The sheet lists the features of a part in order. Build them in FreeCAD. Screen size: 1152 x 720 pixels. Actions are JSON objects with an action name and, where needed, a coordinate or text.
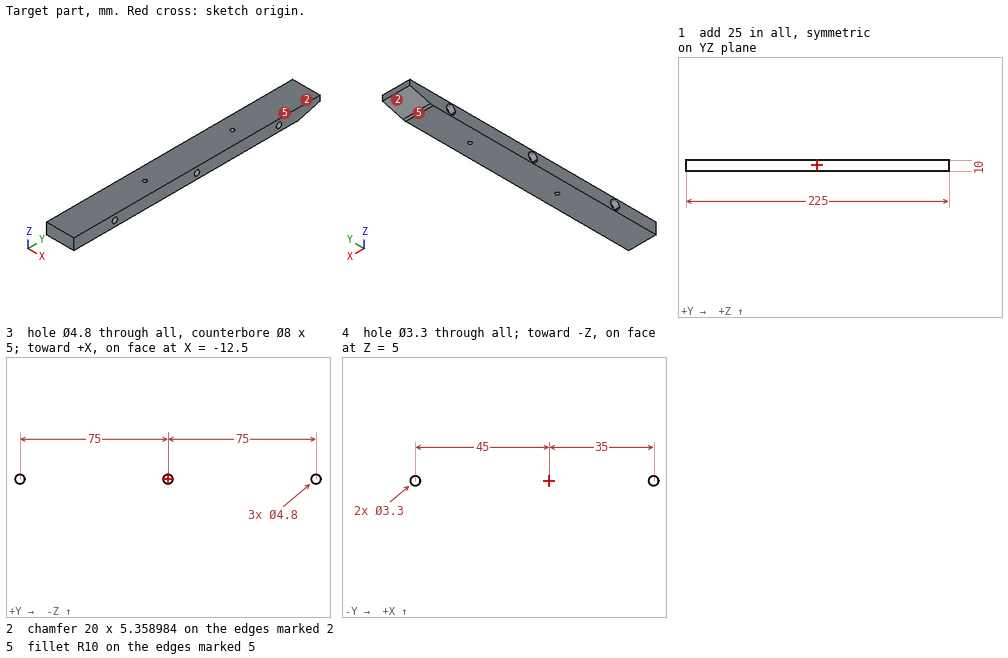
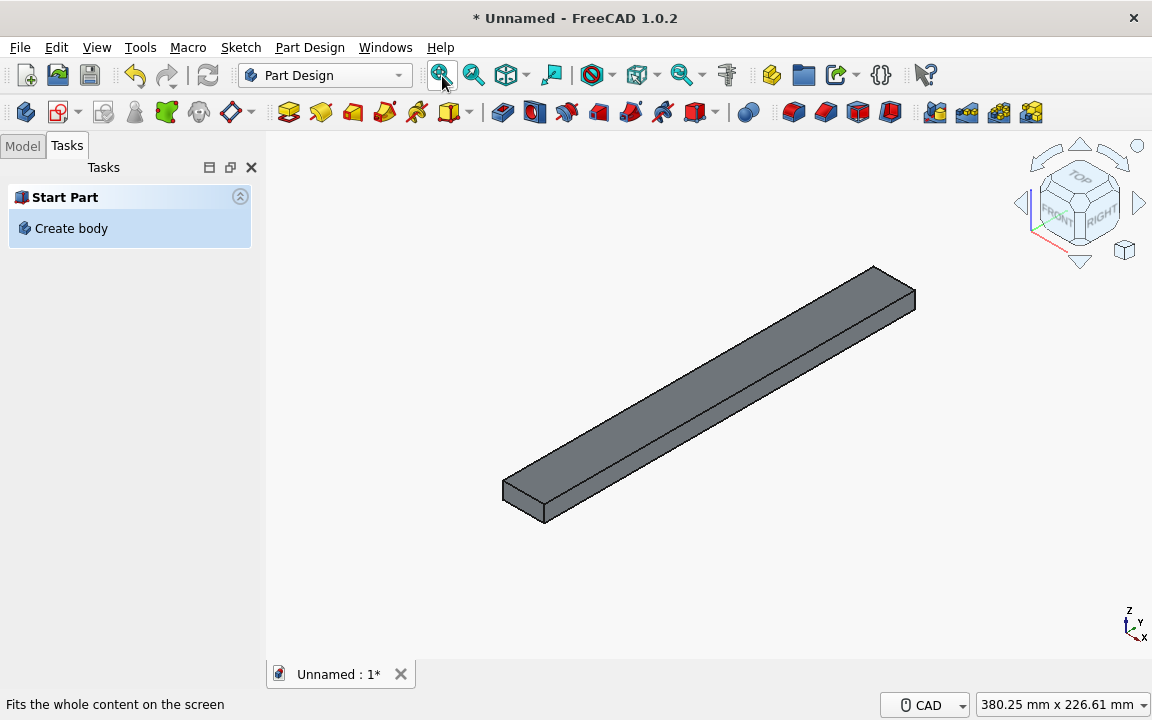
{"action": "key", "text": "2"}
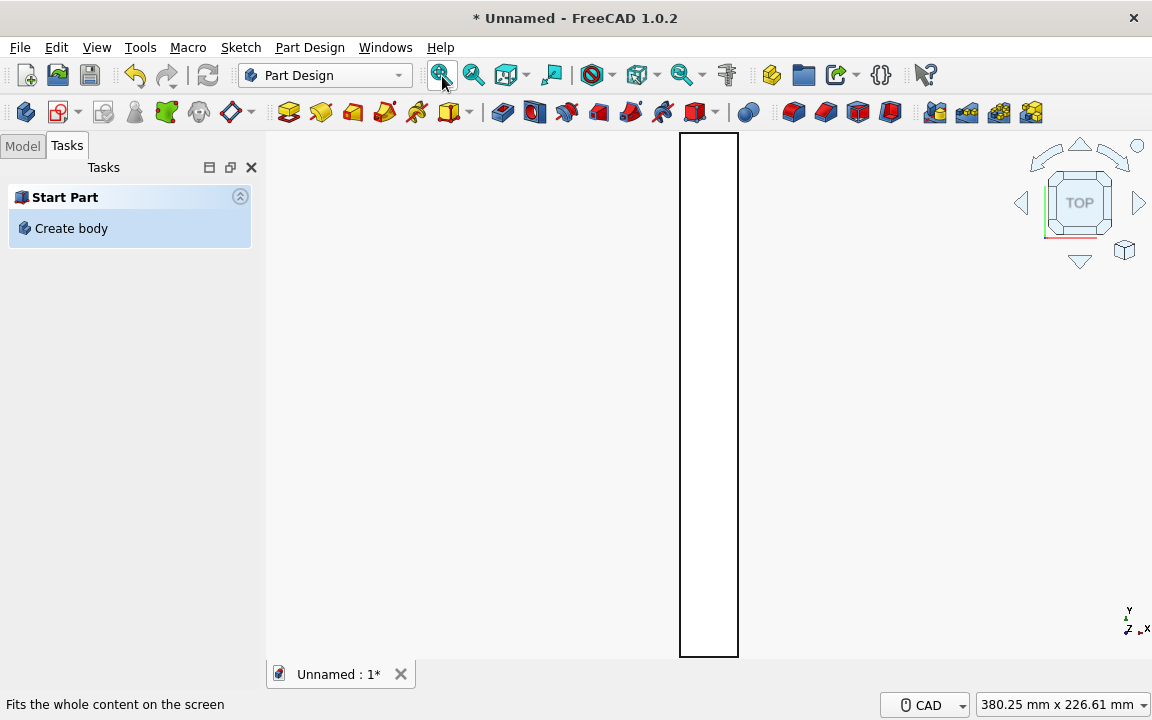
{"action": "key", "text": "1"}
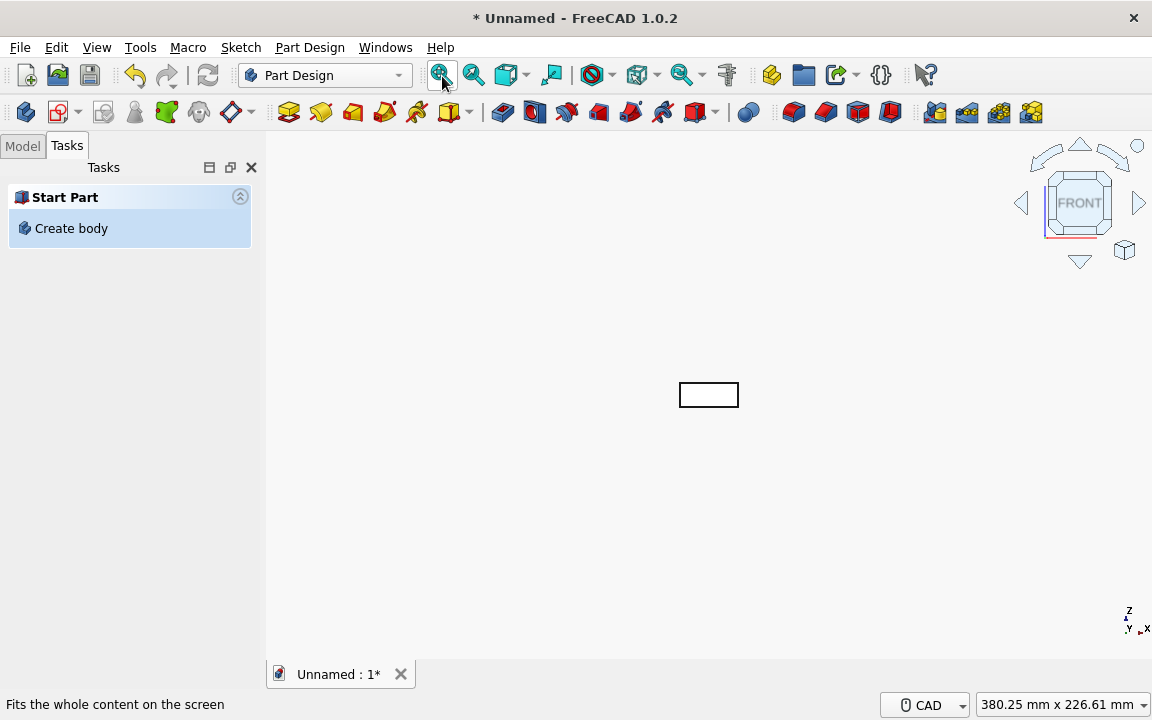
{"action": "left_click", "coordinate": [442, 76]}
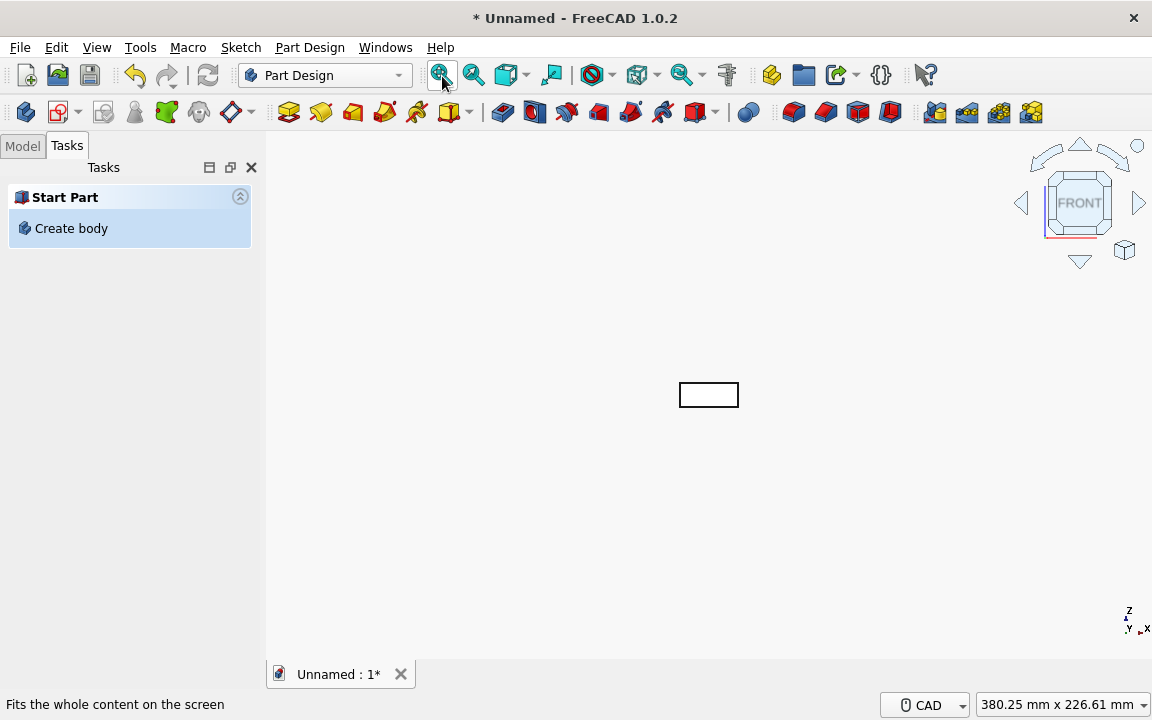
{"action": "key", "text": "3"}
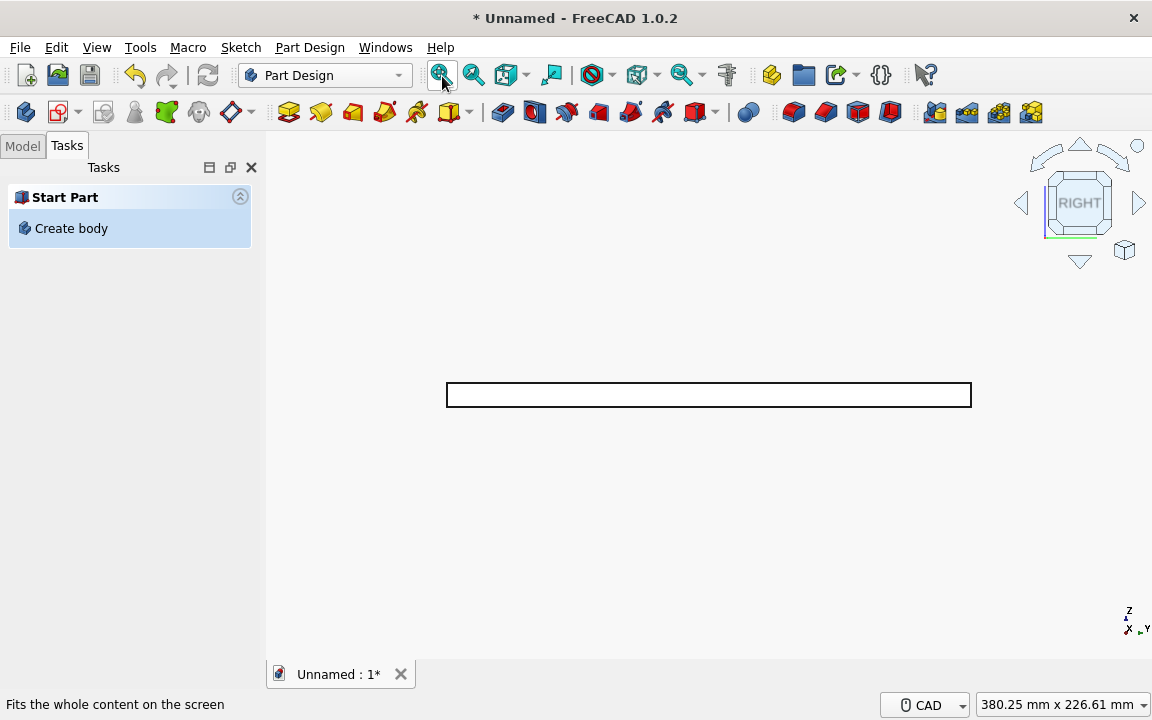
{"action": "key", "text": "5"}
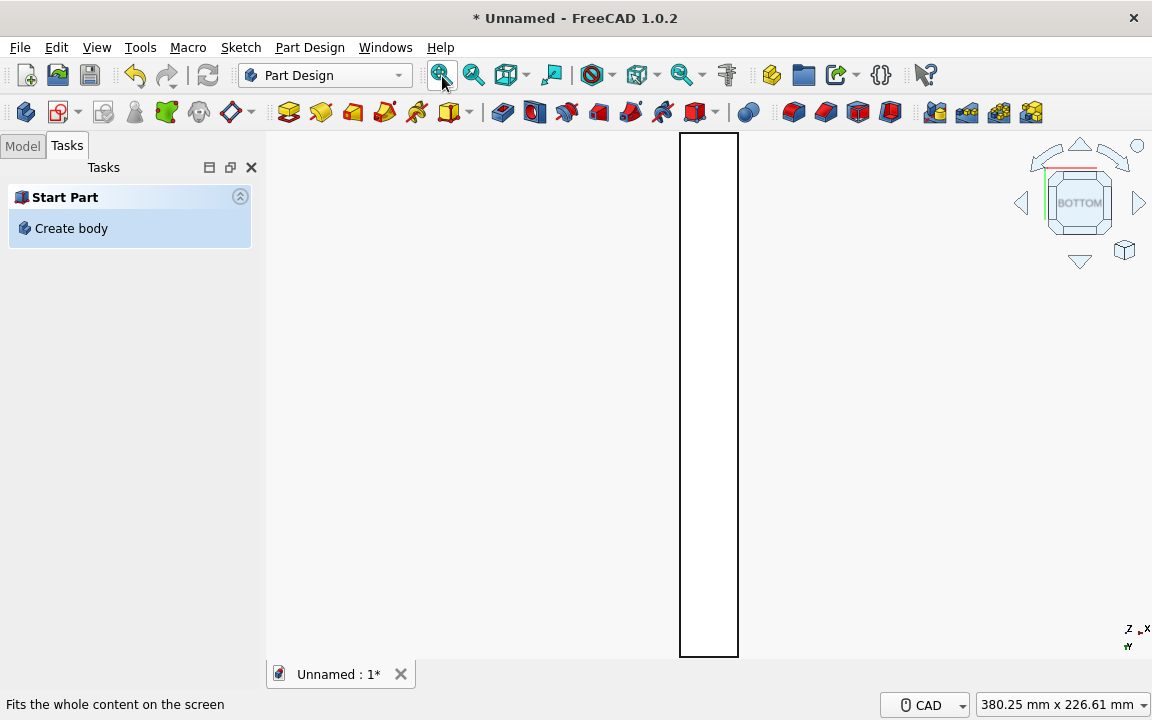
{"action": "key", "text": "4"}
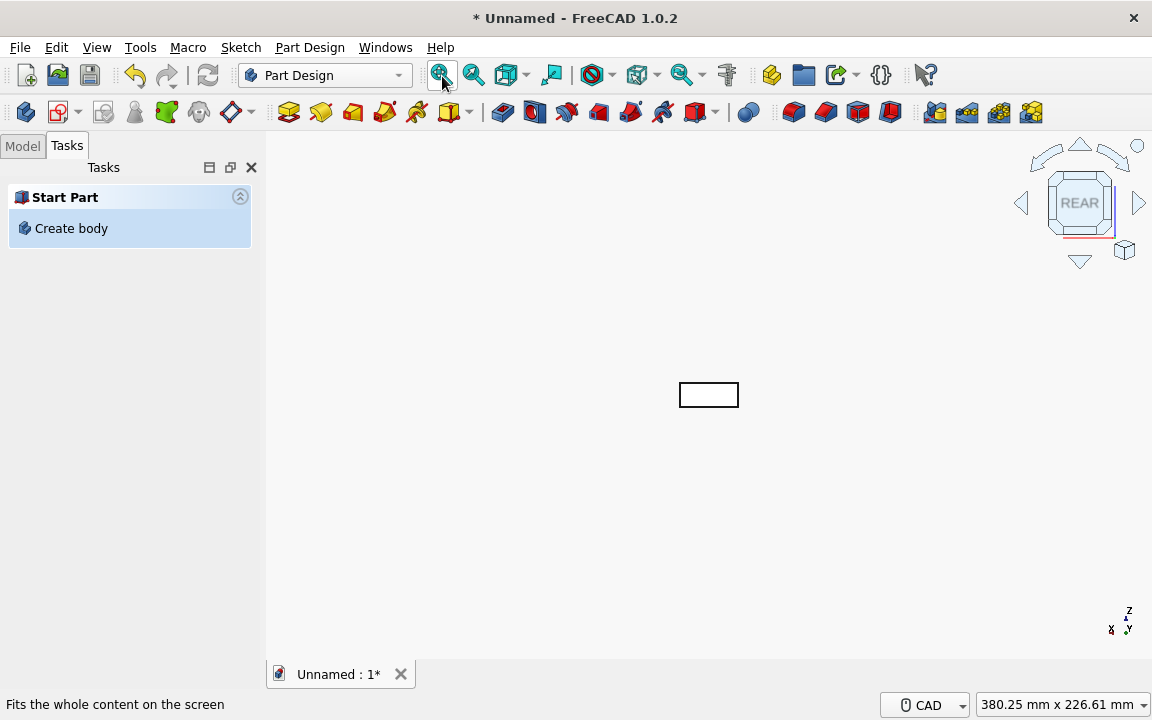
{"action": "left_click", "coordinate": [442, 76]}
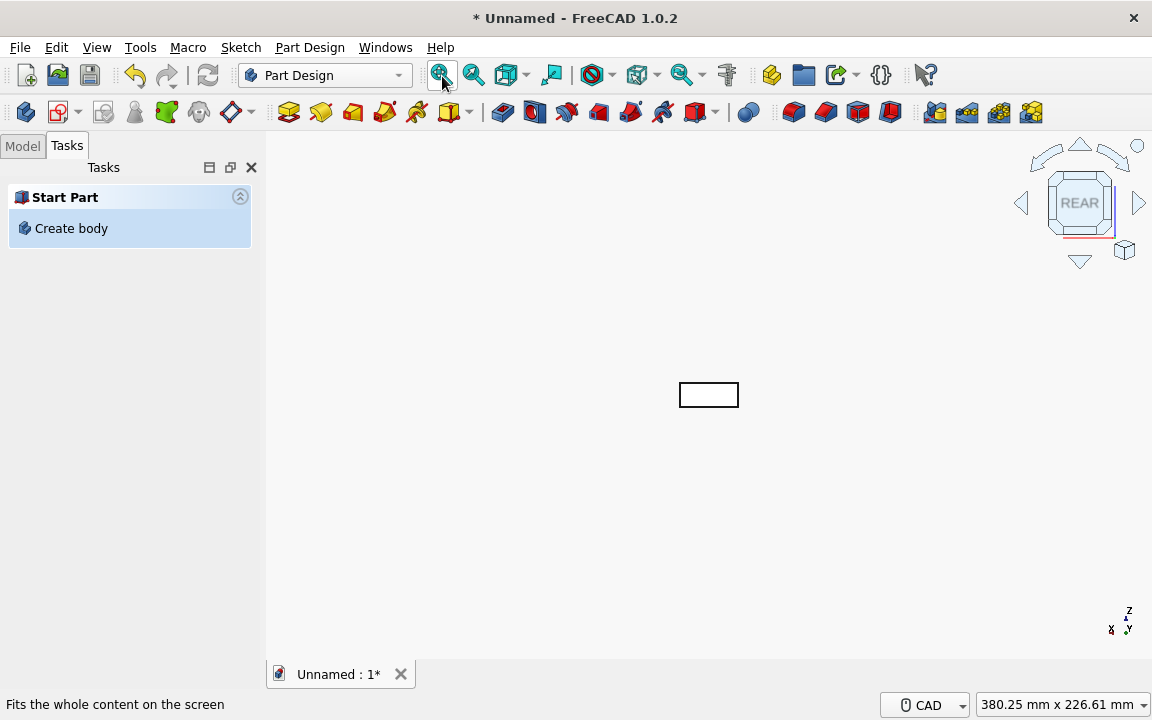
{"action": "left_click", "coordinate": [709, 406]}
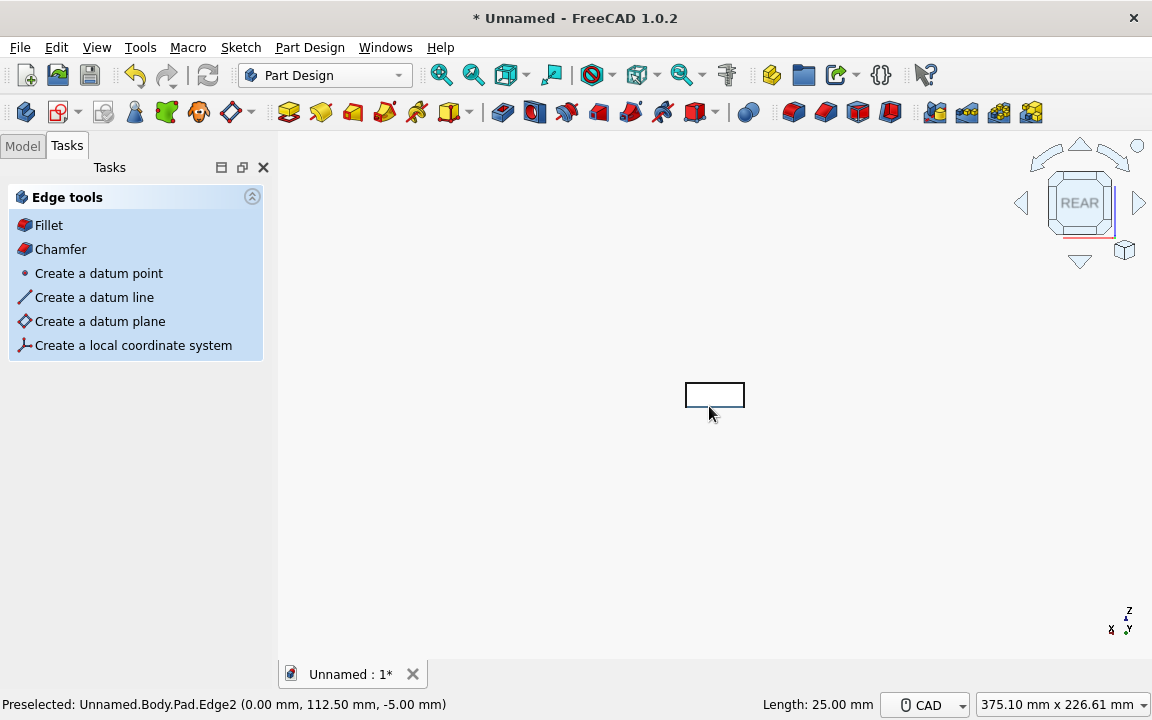
{"action": "left_click", "coordinate": [826, 112]}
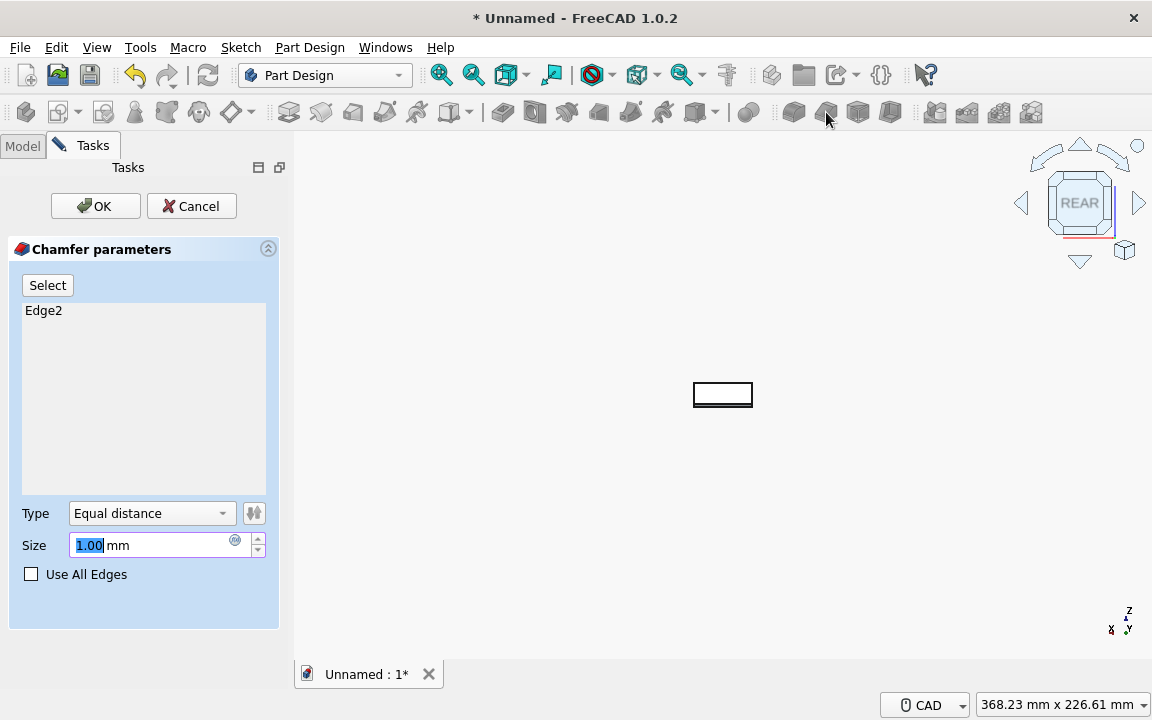
{"action": "type", "text": "20"}
{"action": "key", "text": "Tab"}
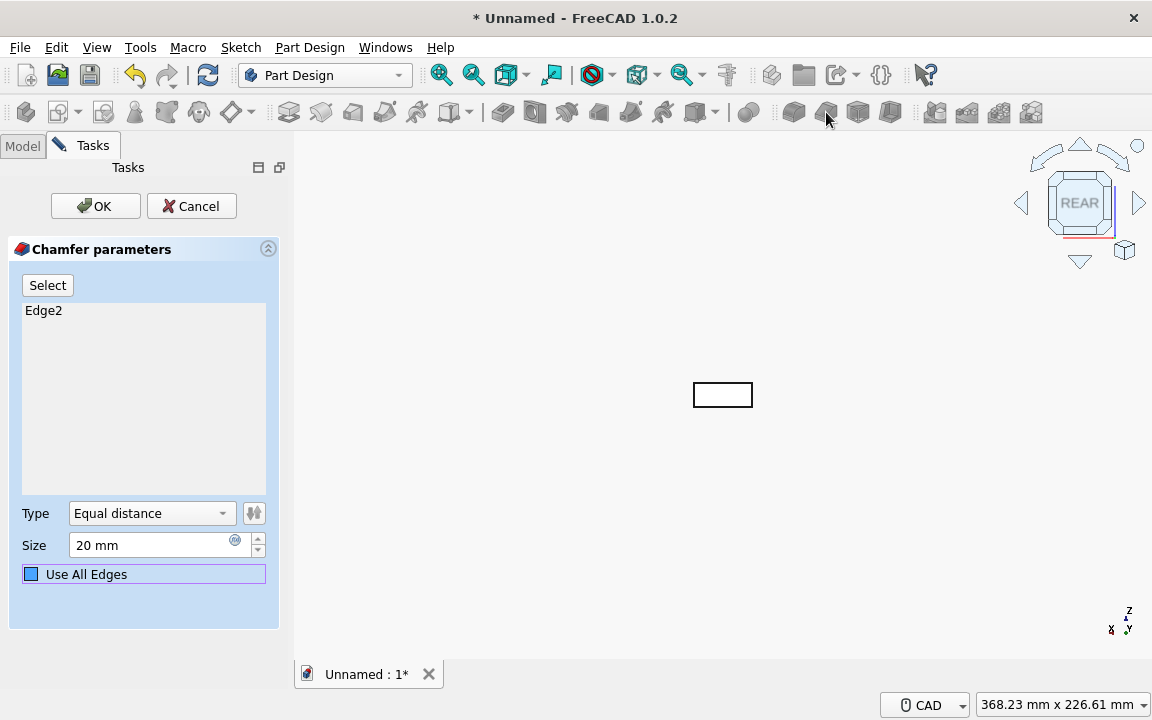
{"action": "left_click", "coordinate": [153, 514]}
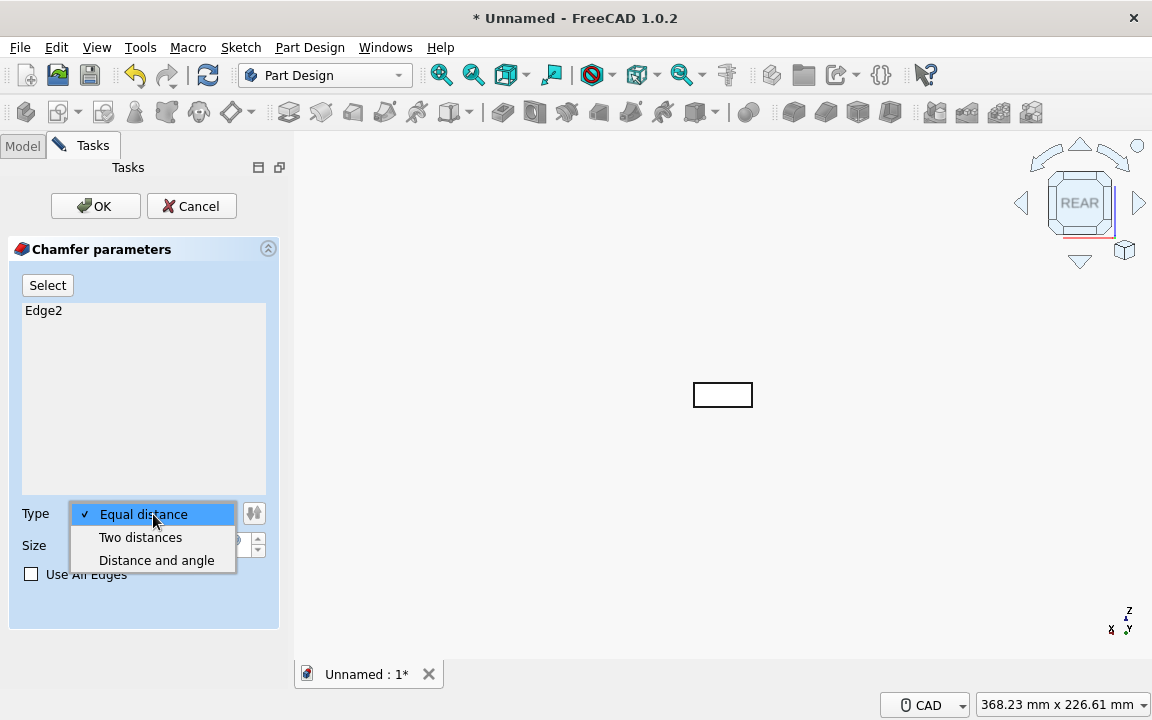
{"action": "left_click", "coordinate": [152, 538]}